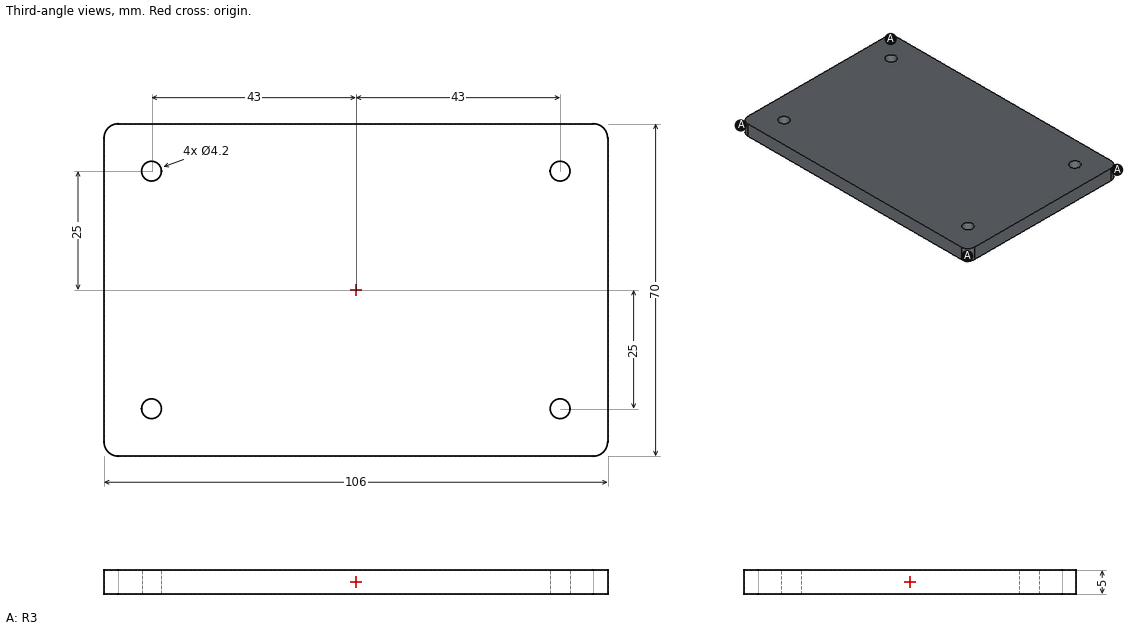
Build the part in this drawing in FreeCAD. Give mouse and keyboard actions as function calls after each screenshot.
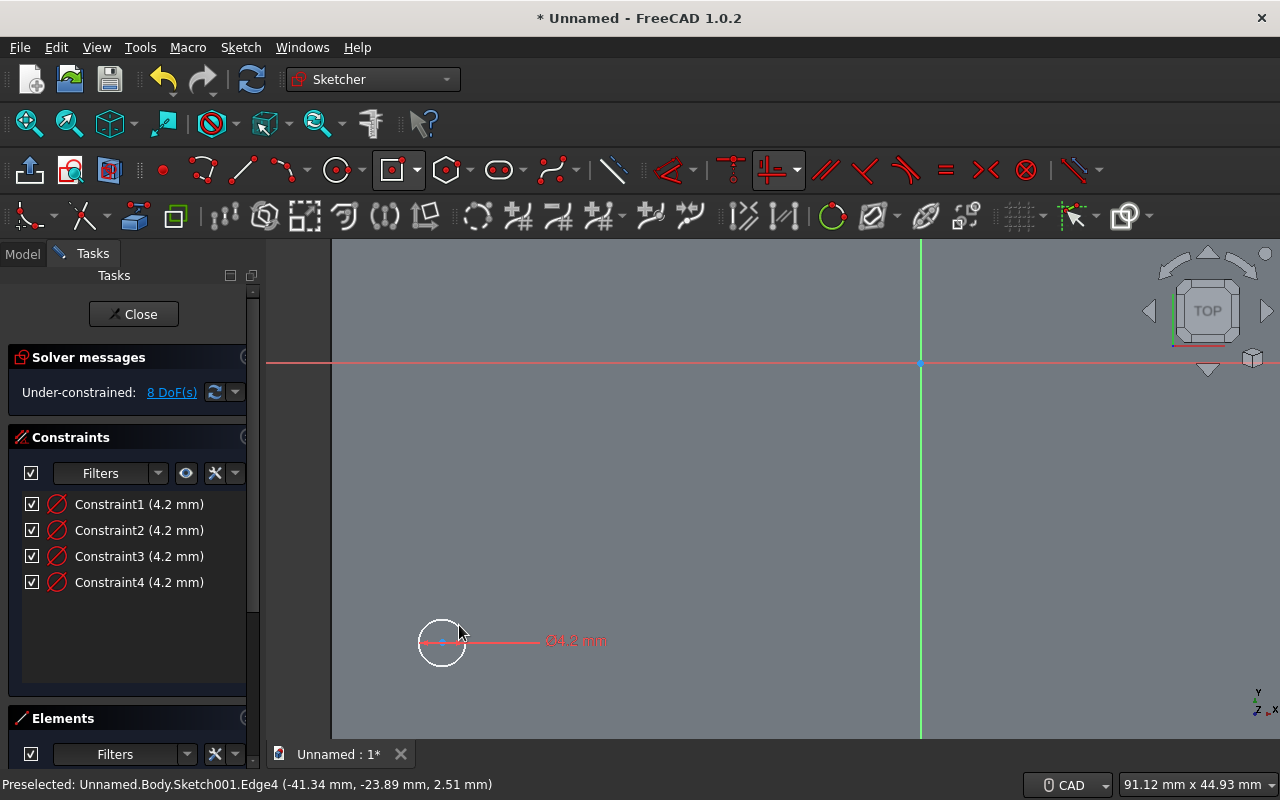
scroll(441, 642, down, 3)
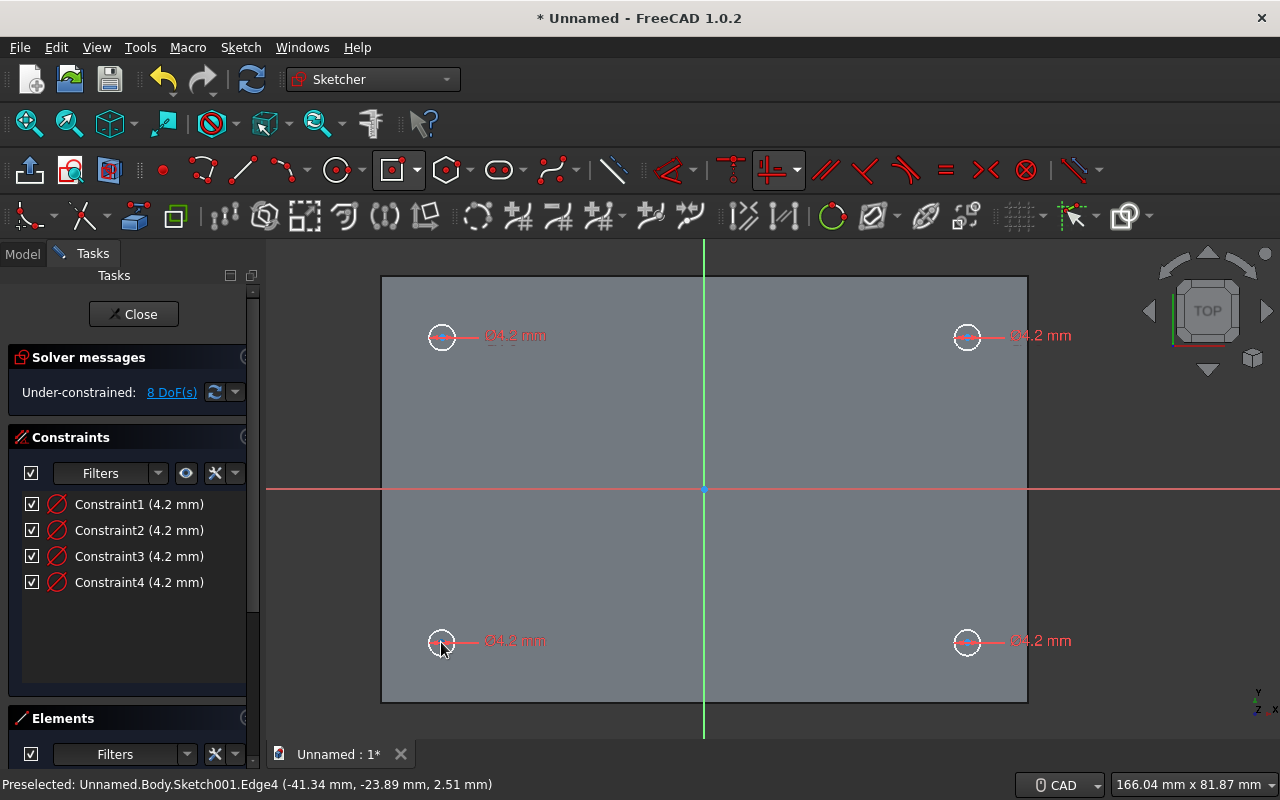
click(442, 338)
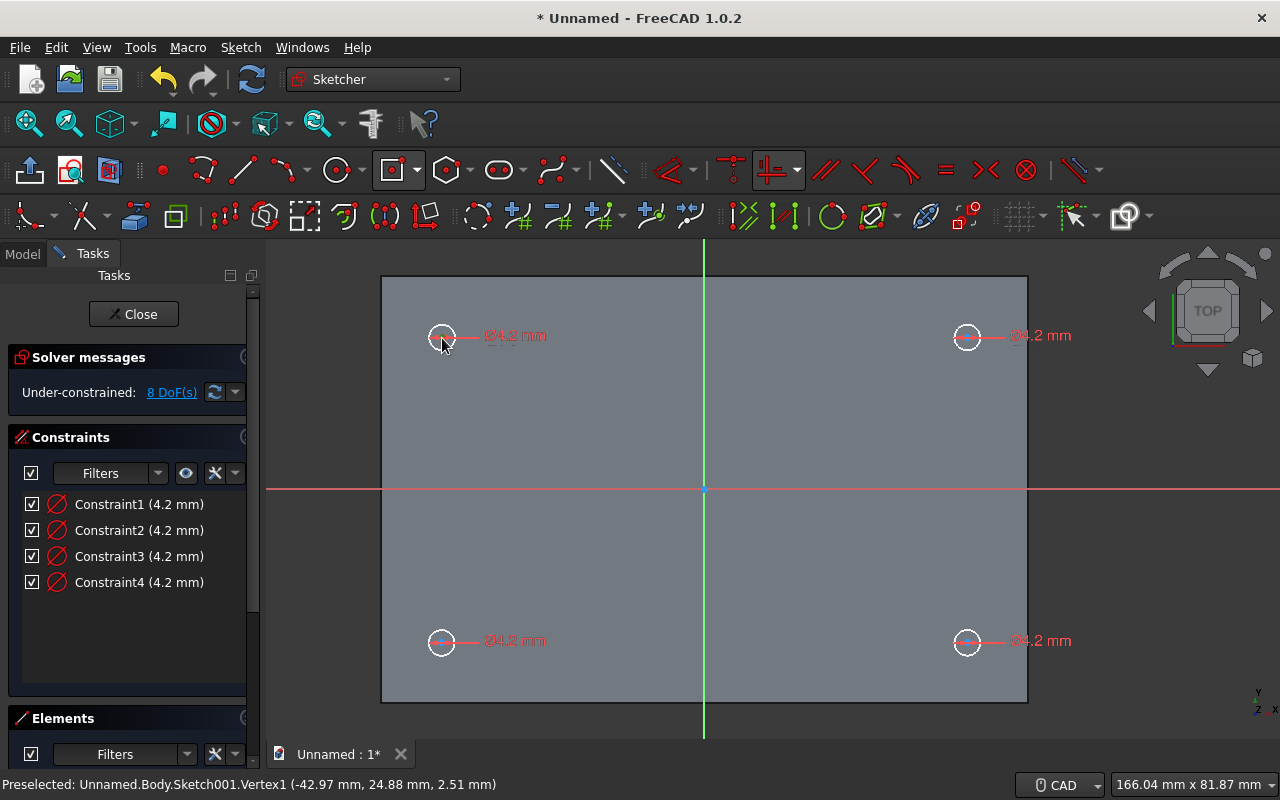
click(967, 338)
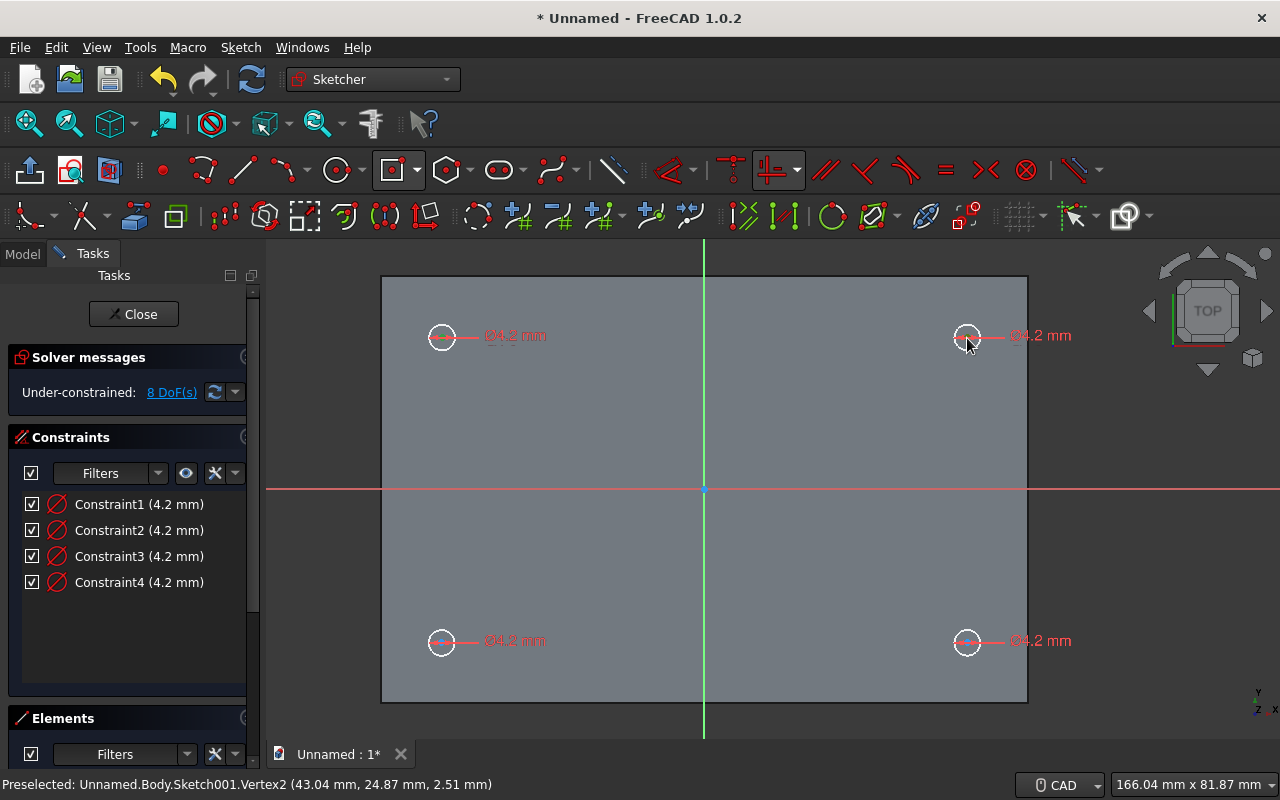
key(h)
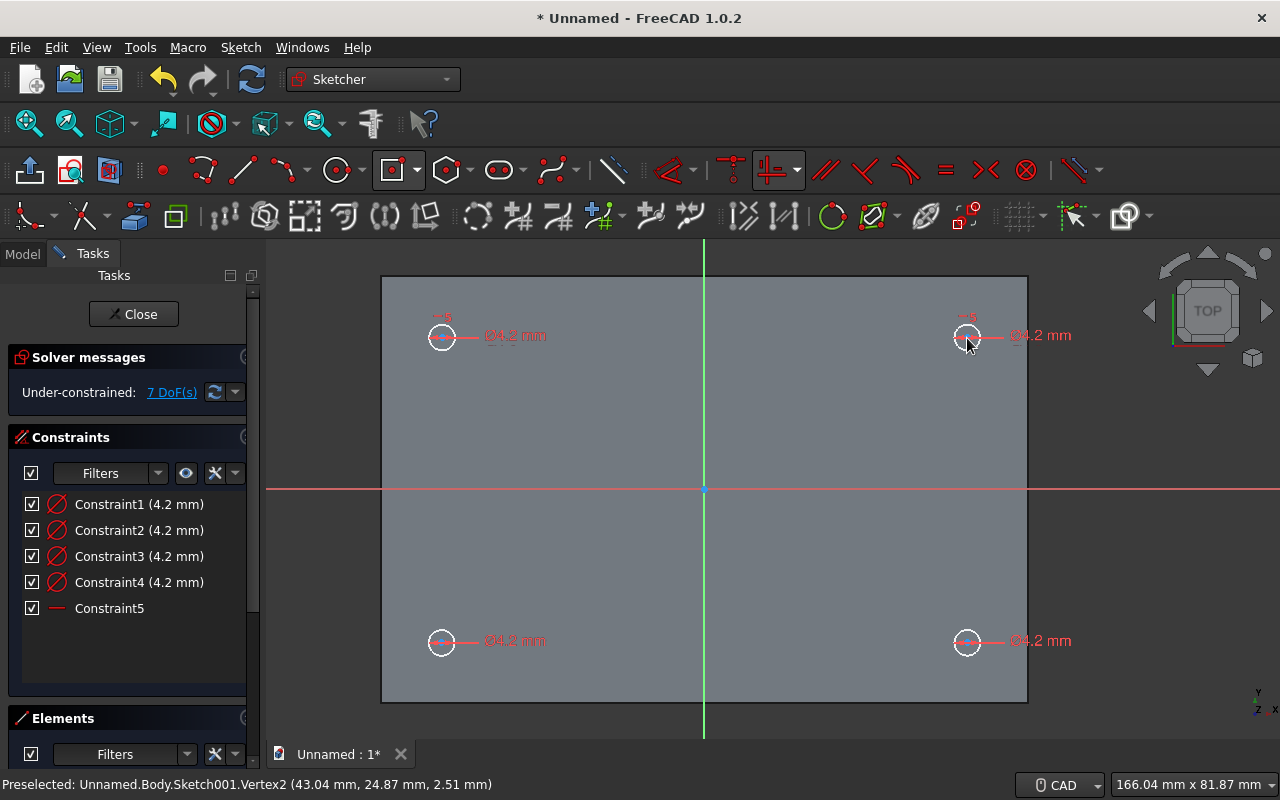
click(967, 338)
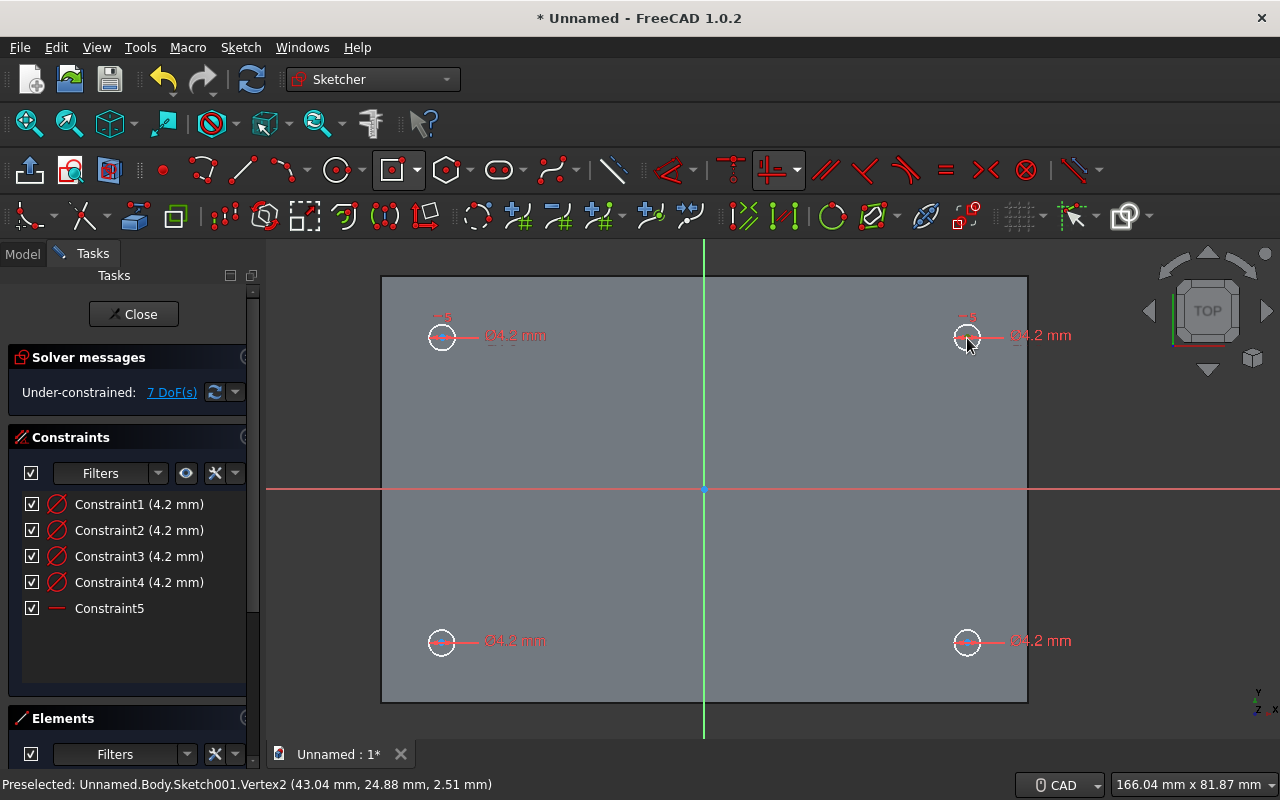
click(967, 643)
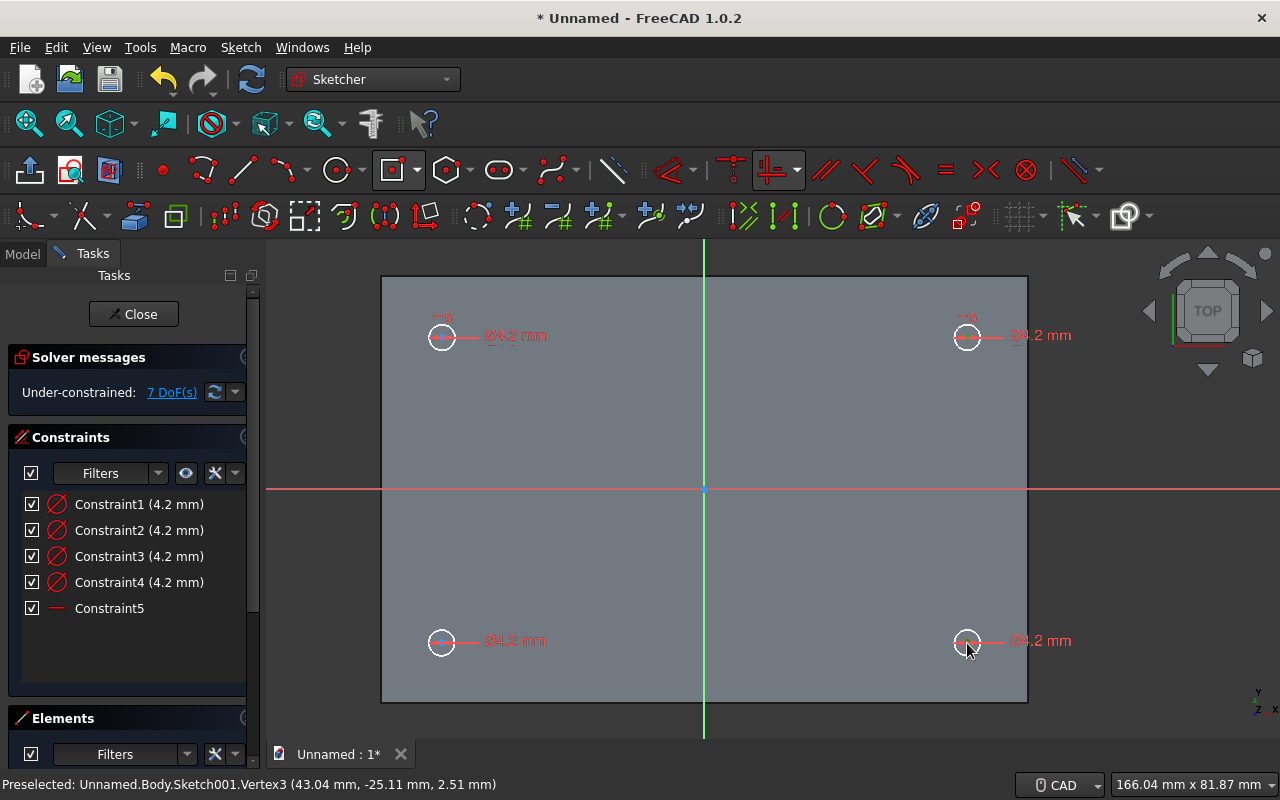
key(v)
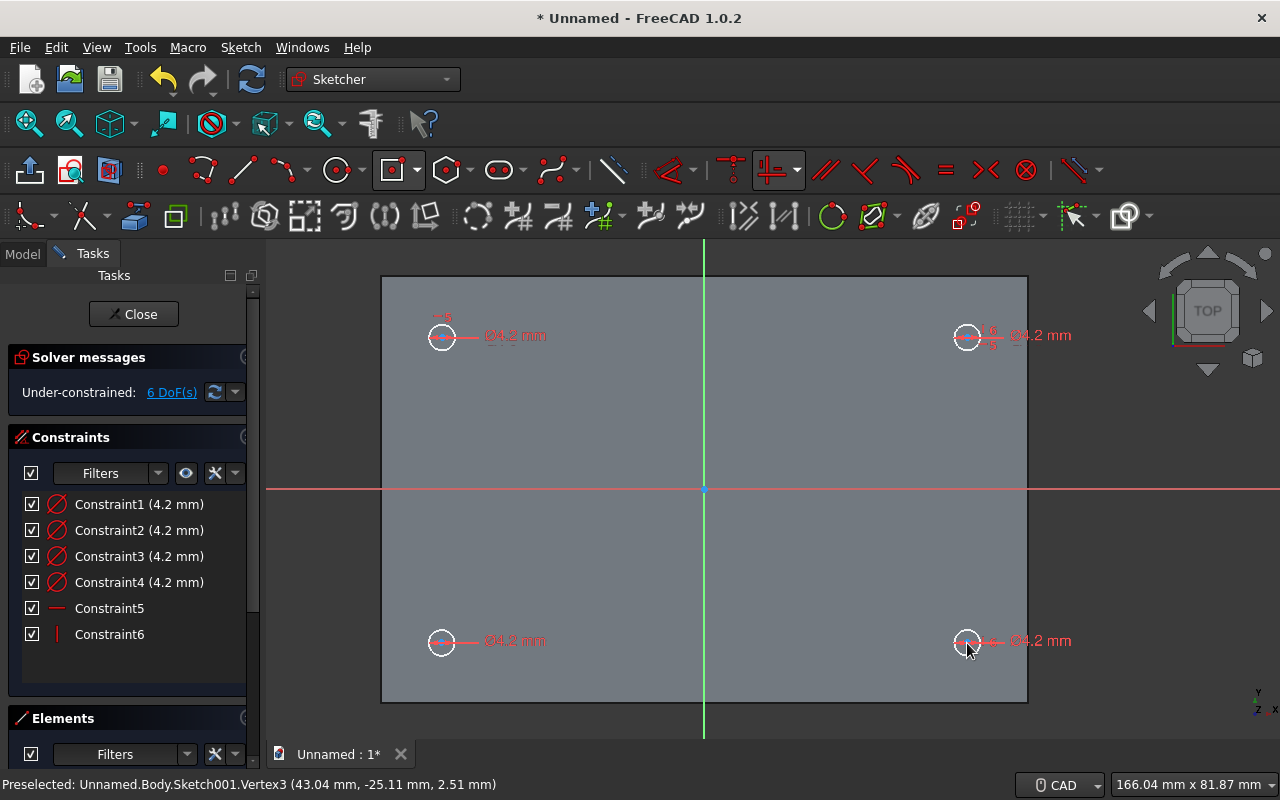
click(442, 338)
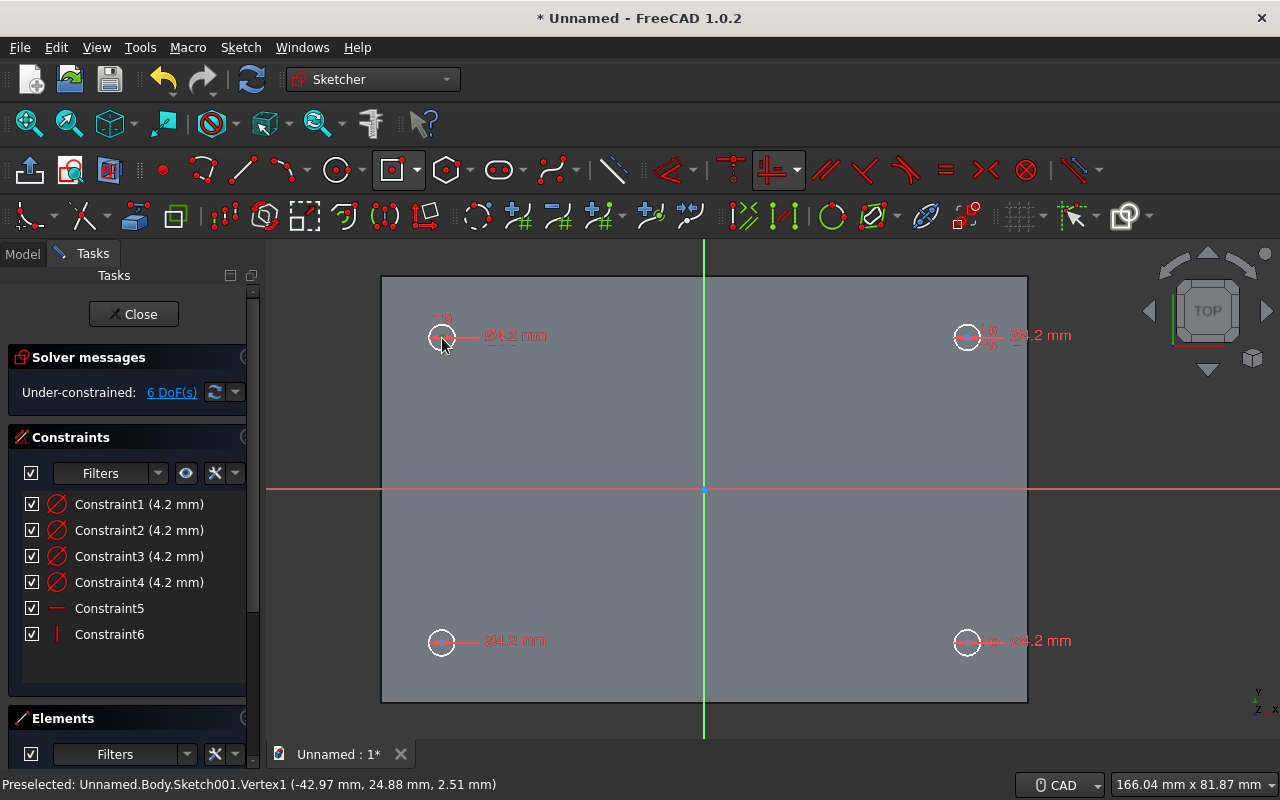
click(442, 643)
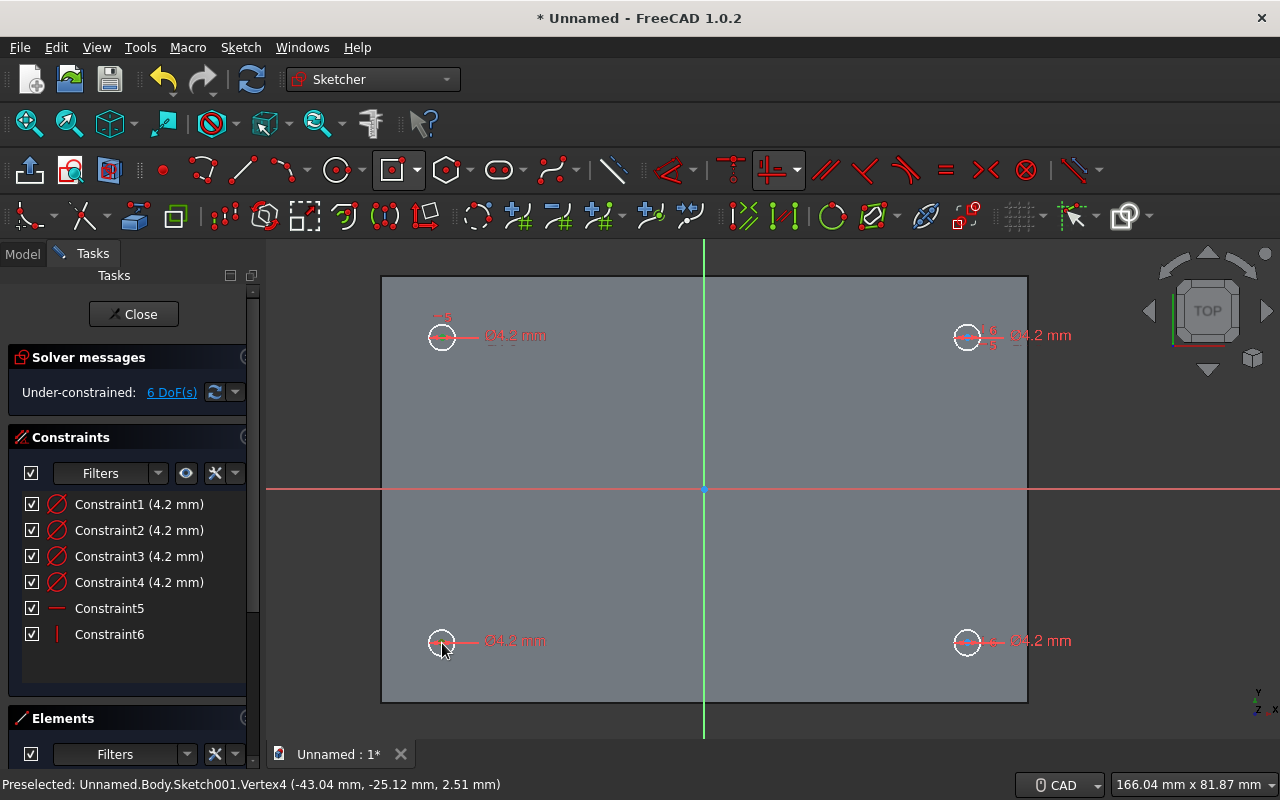
key(v)